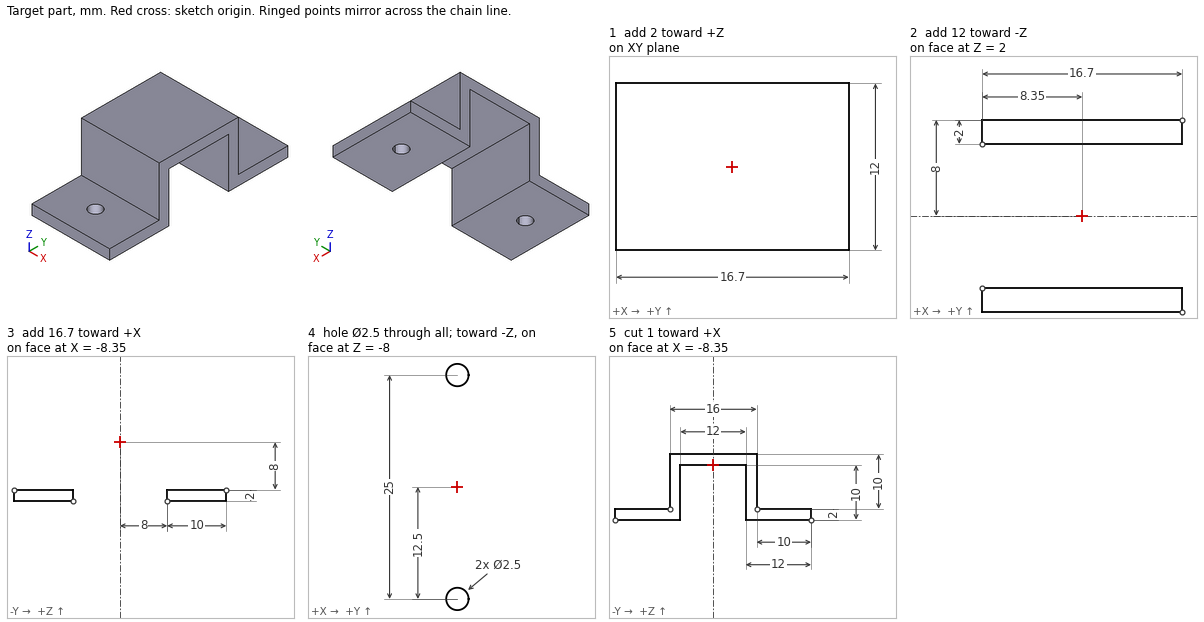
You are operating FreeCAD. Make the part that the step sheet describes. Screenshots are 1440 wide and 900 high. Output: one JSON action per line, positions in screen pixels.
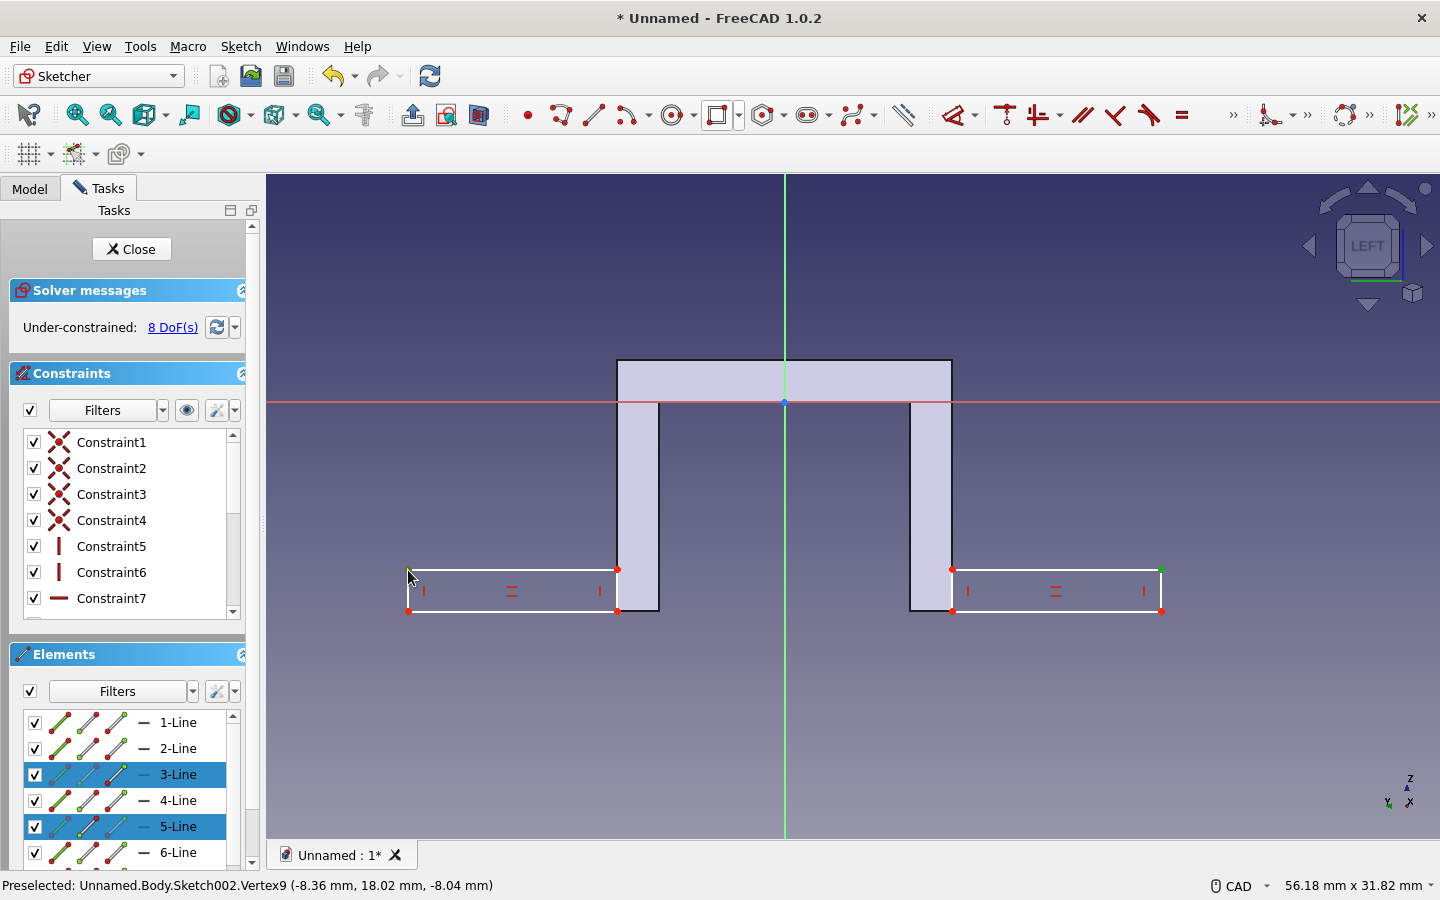
{"action": "left_click", "coordinate": [785, 768]}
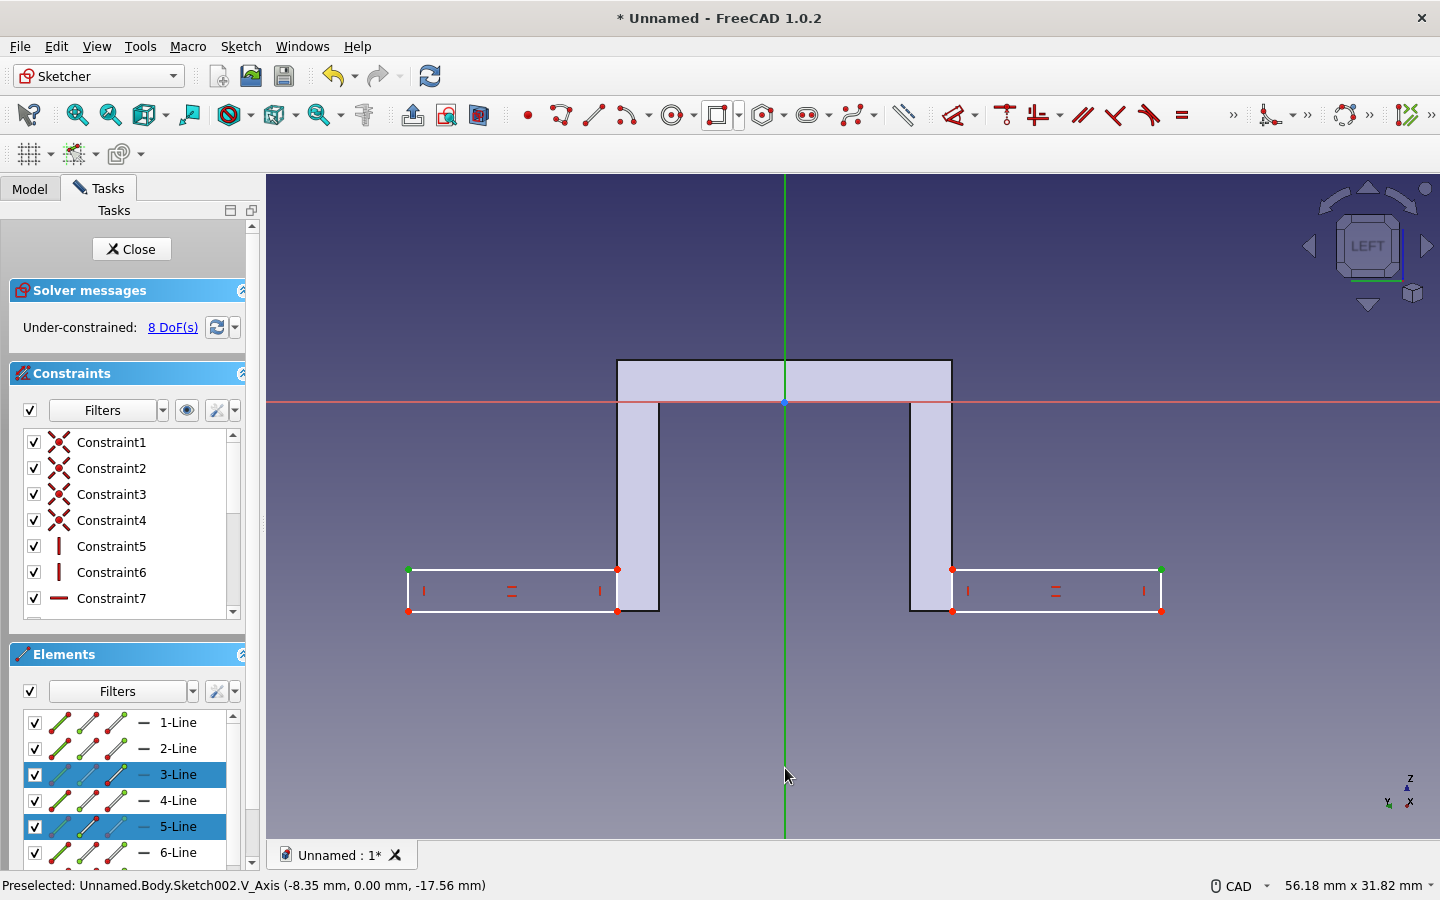
{"action": "key", "text": "s"}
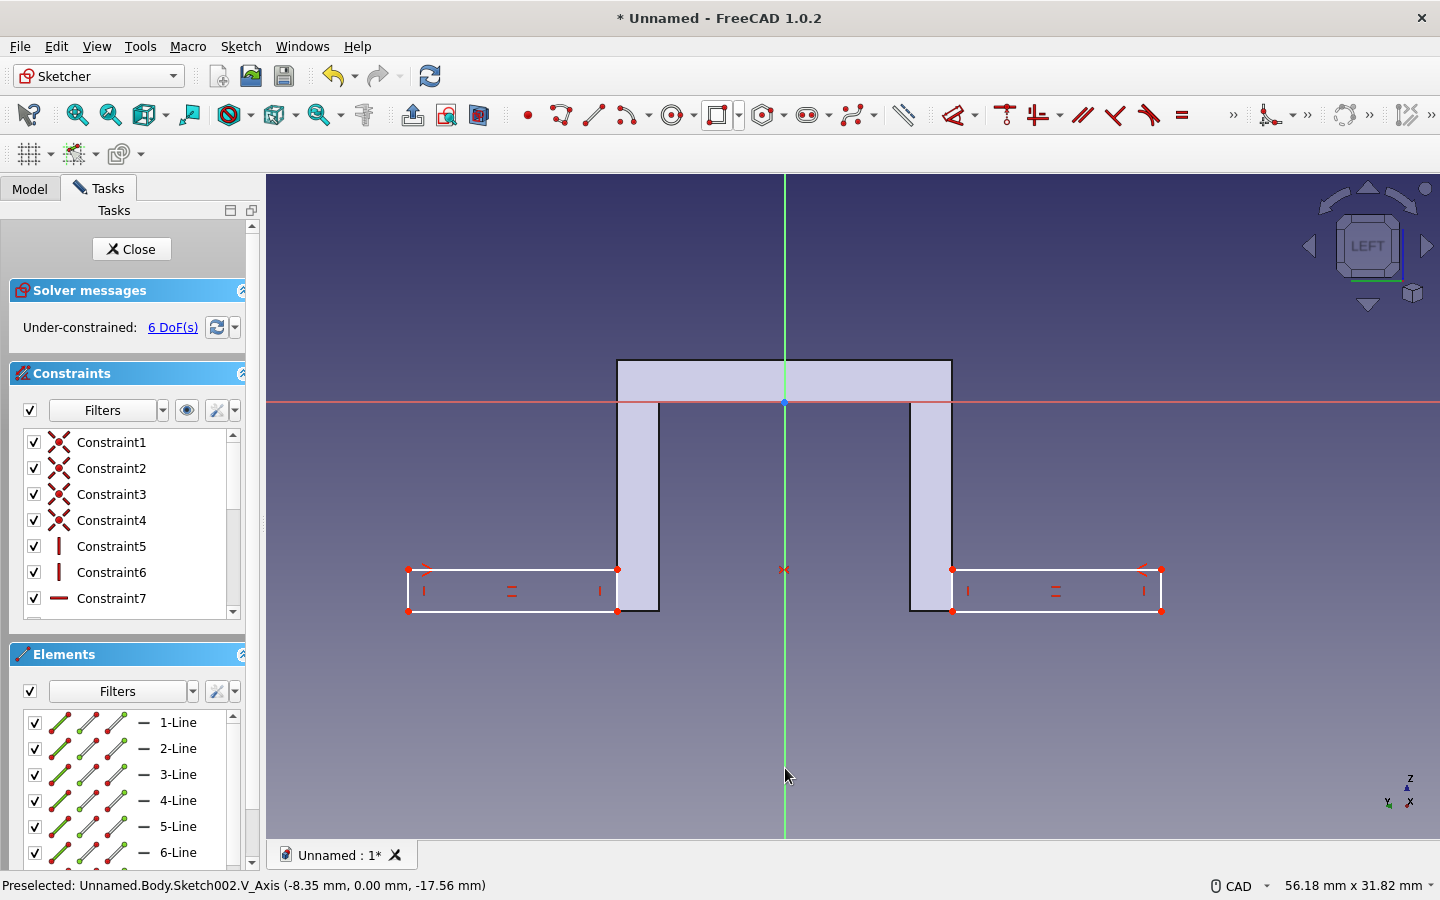
{"action": "left_click", "coordinate": [952, 612]}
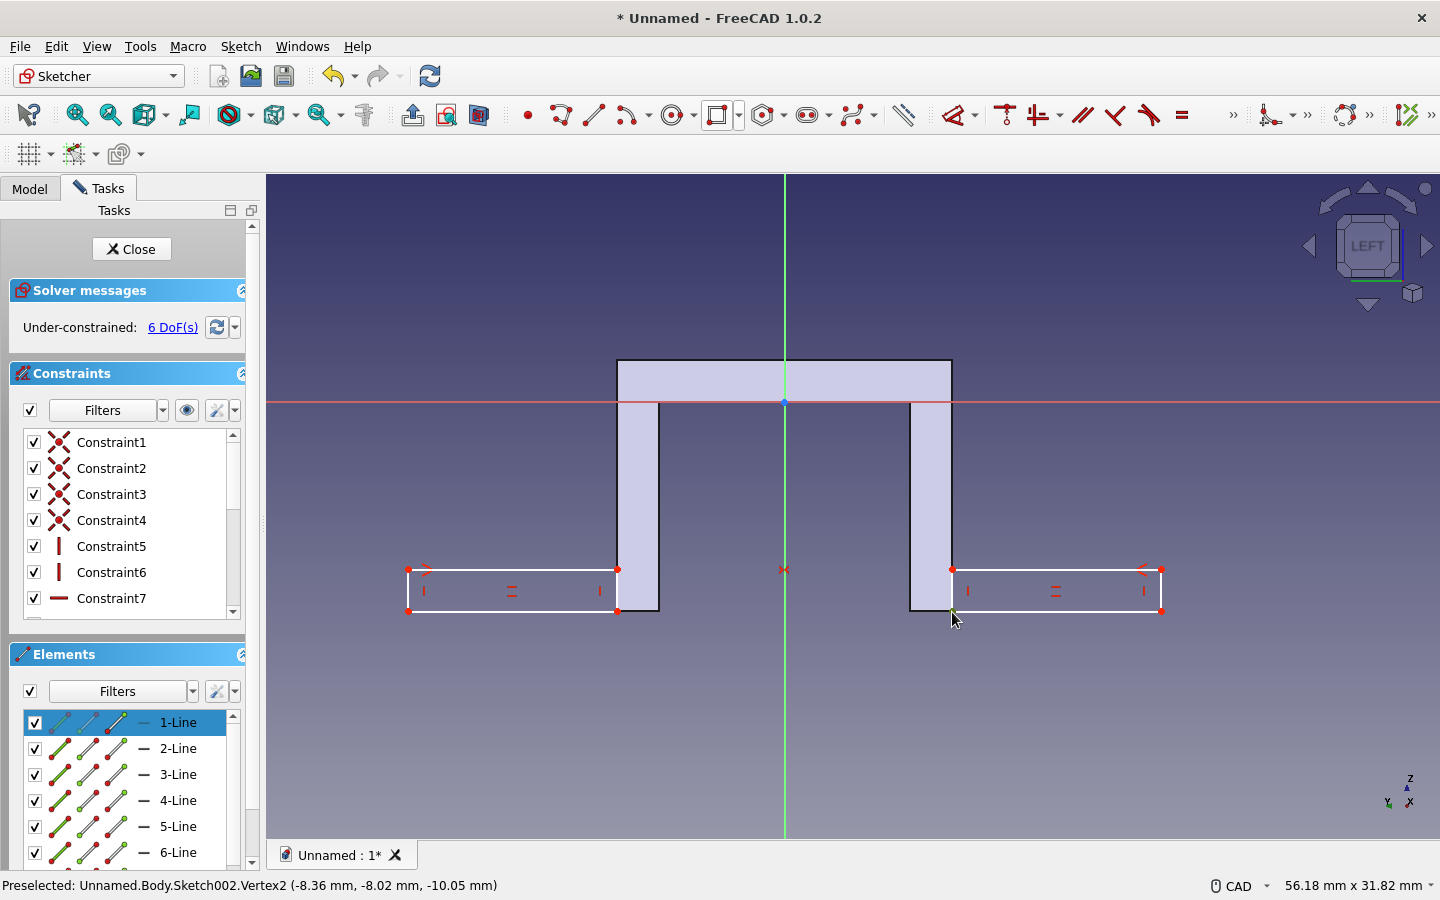
{"action": "left_click", "coordinate": [617, 612]}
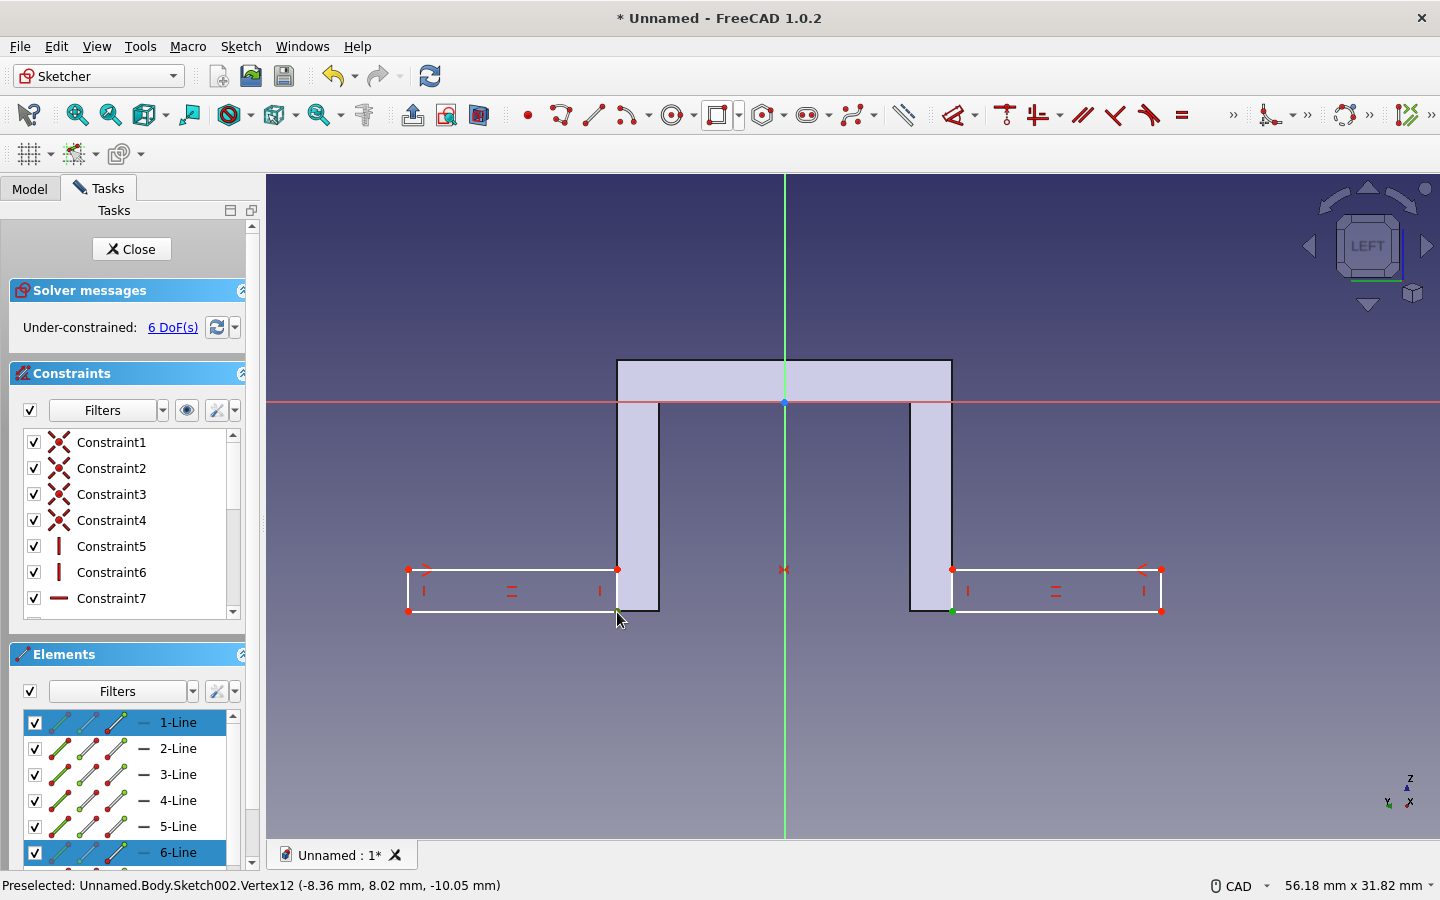
{"action": "left_click", "coordinate": [785, 768]}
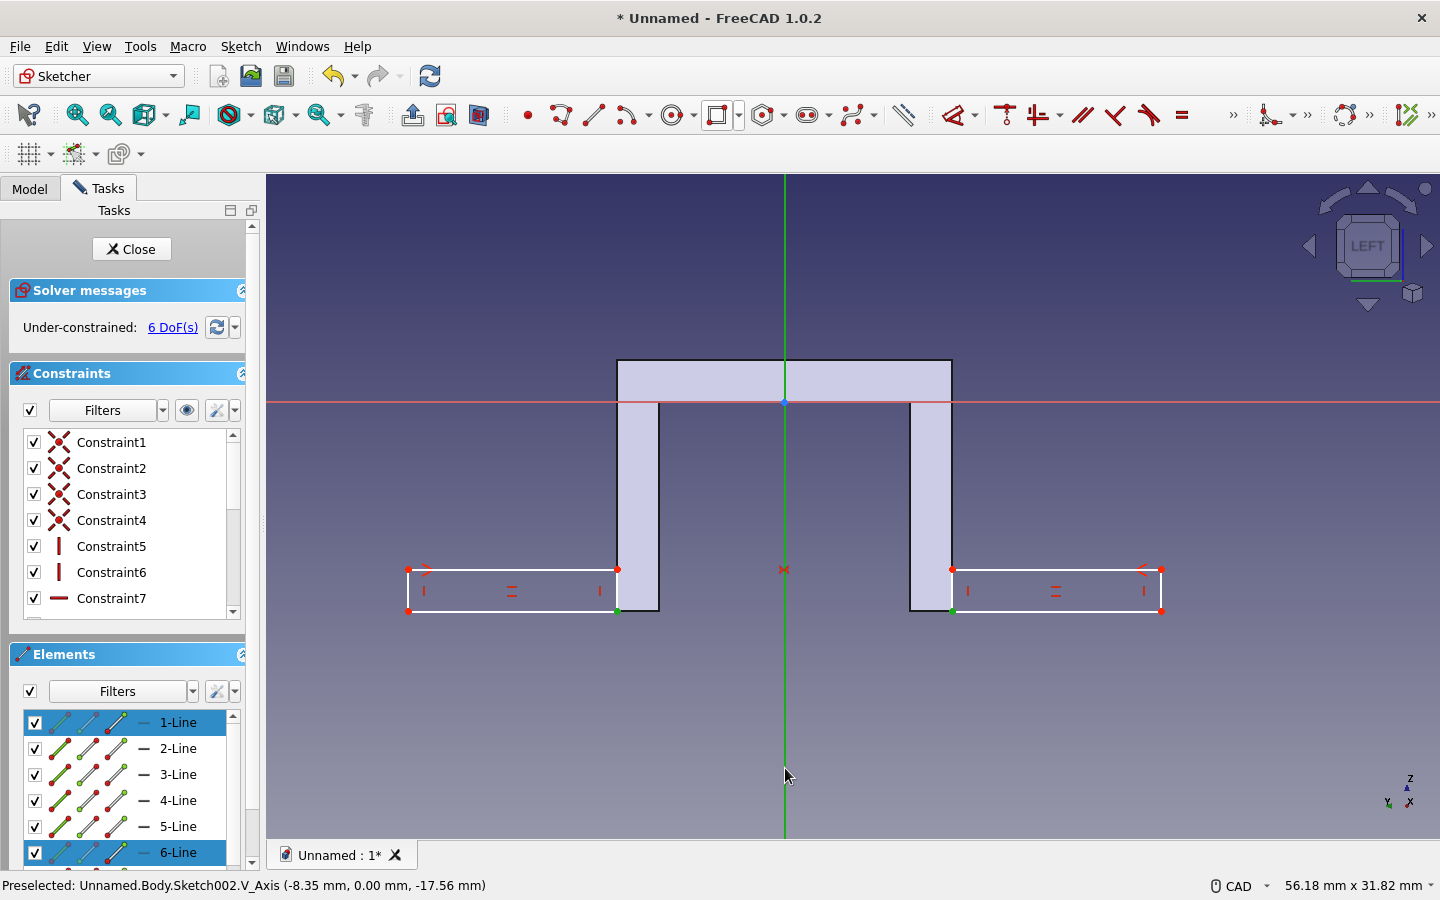
{"action": "key", "text": "s"}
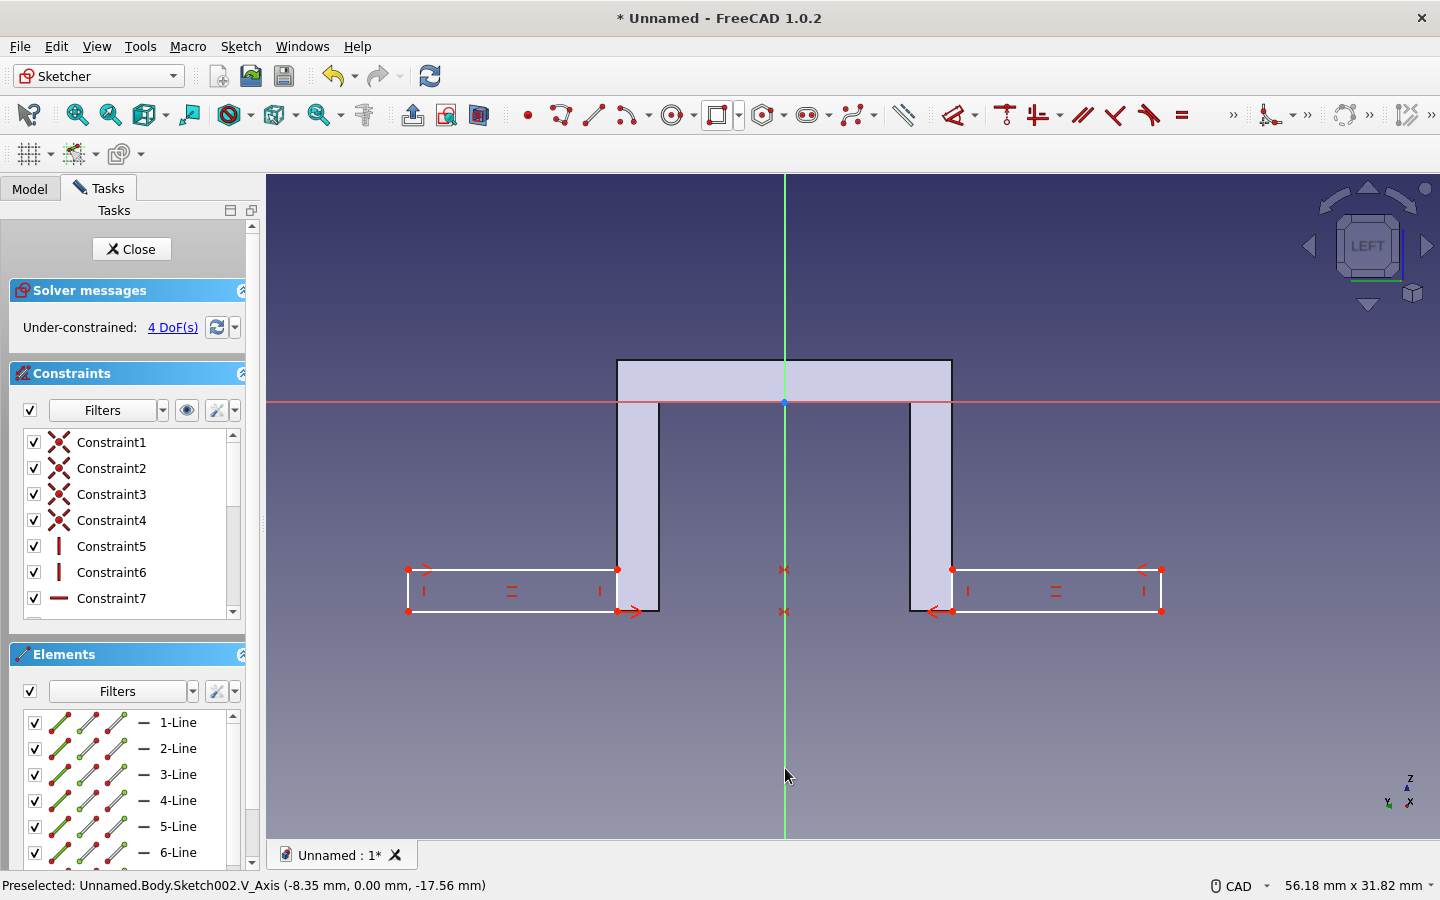
{"action": "key", "text": "d"}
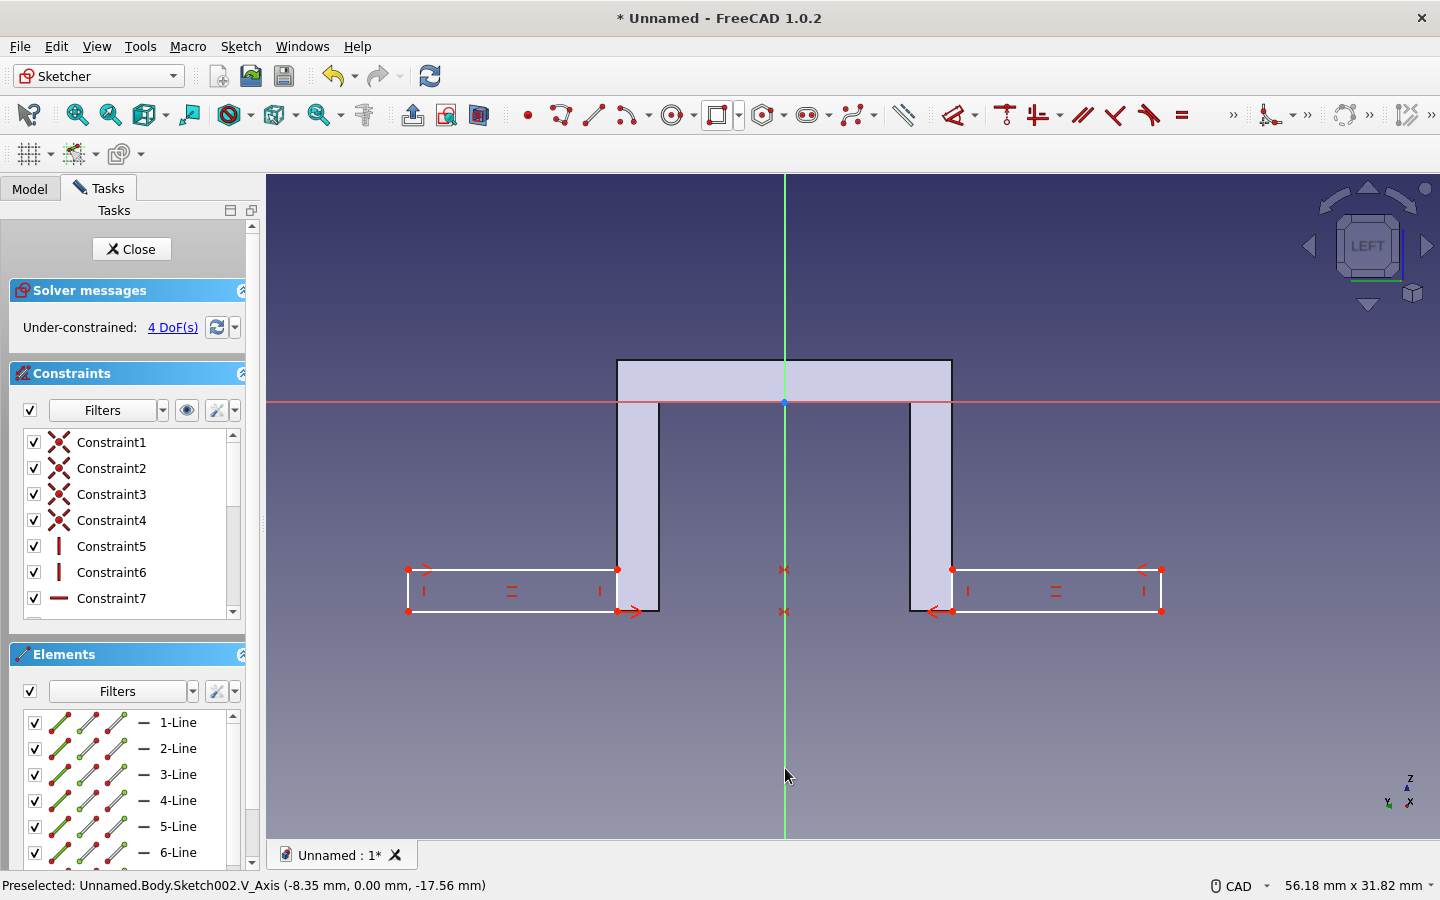
{"action": "left_click", "coordinate": [952, 583]}
{"action": "left_click", "coordinate": [986, 591]}